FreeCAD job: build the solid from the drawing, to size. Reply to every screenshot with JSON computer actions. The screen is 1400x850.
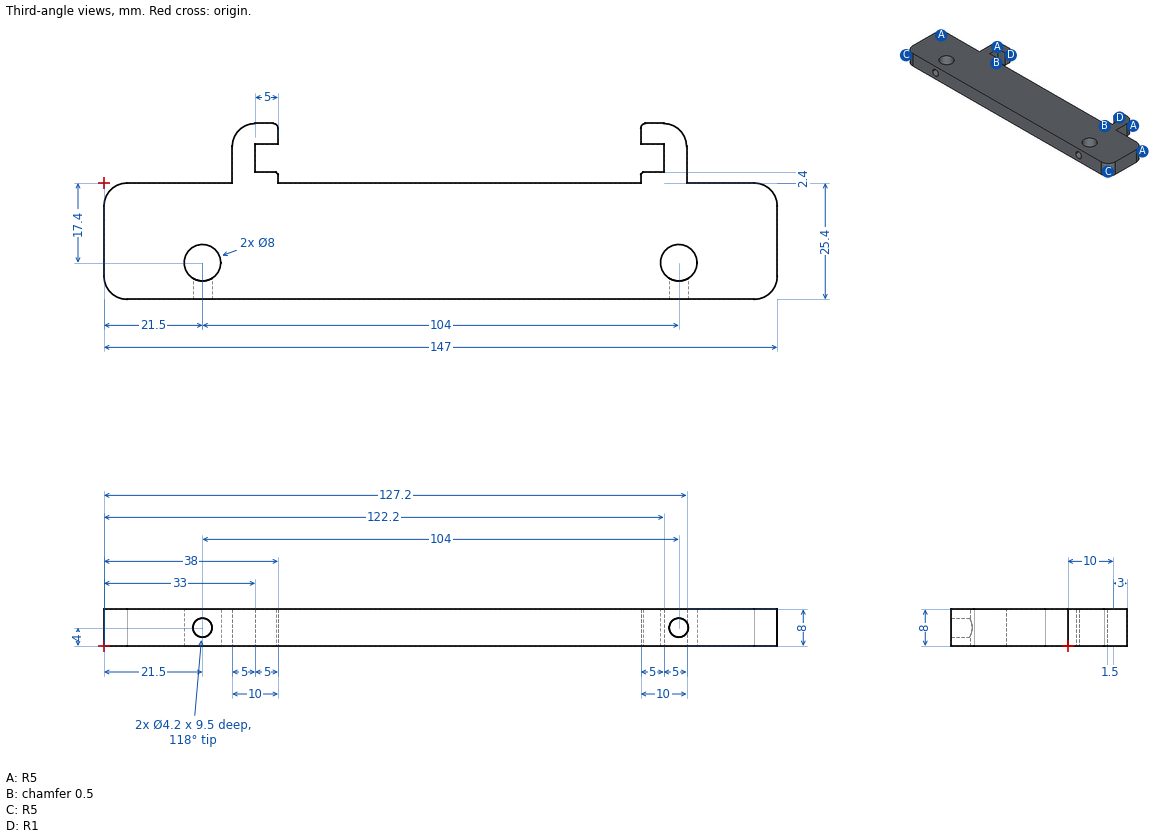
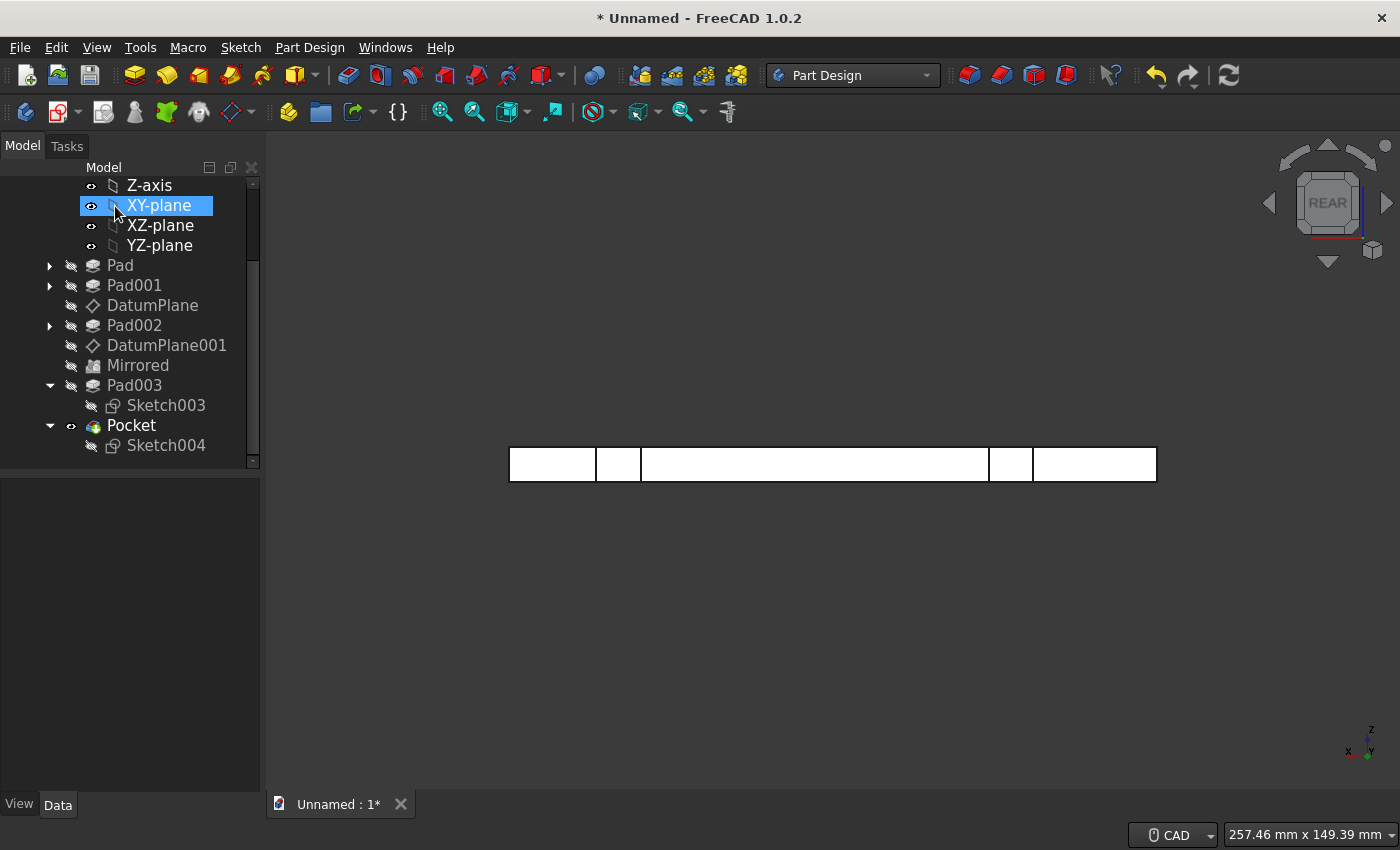
{"action": "left_click", "coordinate": [619, 463]}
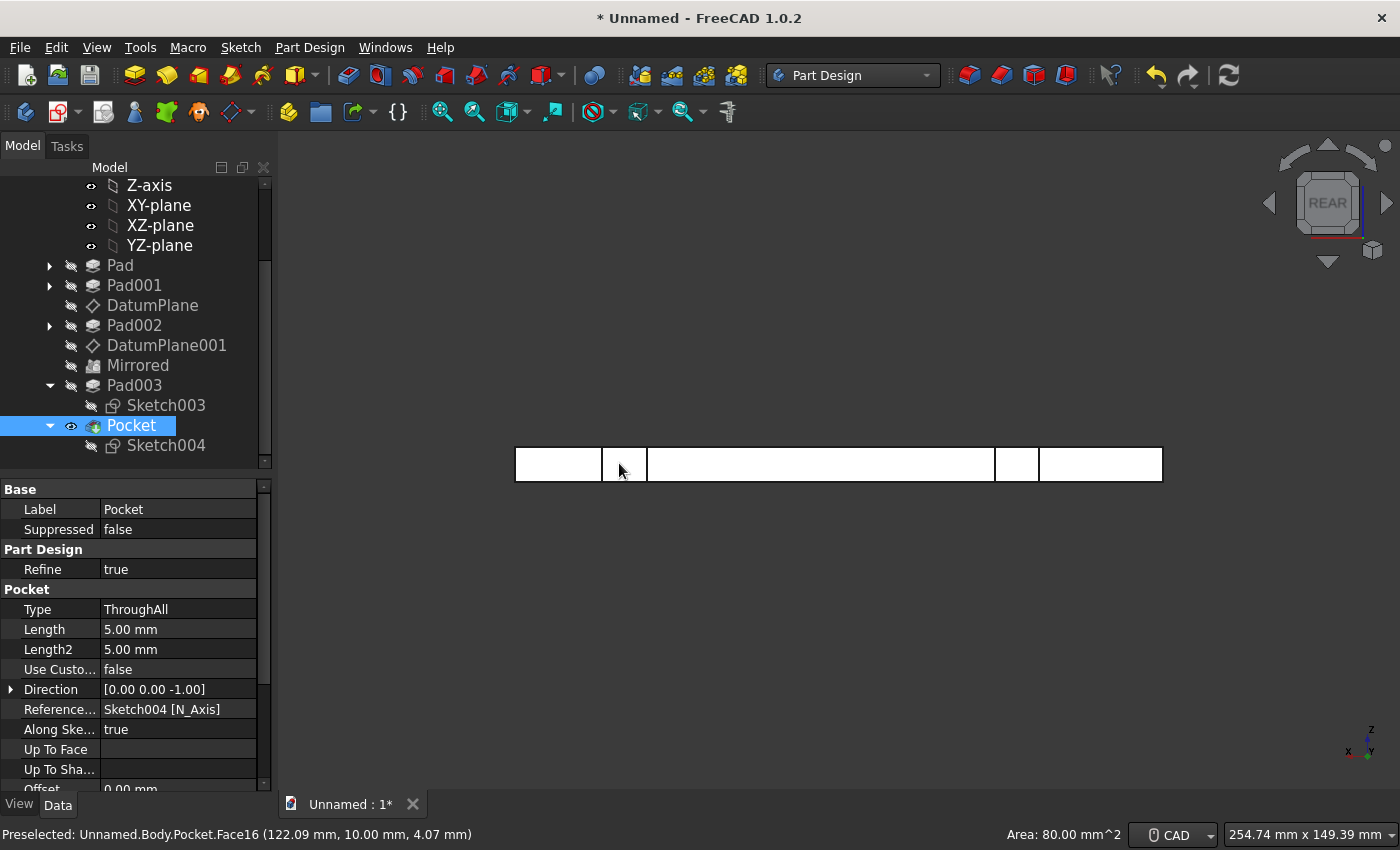
{"action": "left_click", "coordinate": [58, 112]}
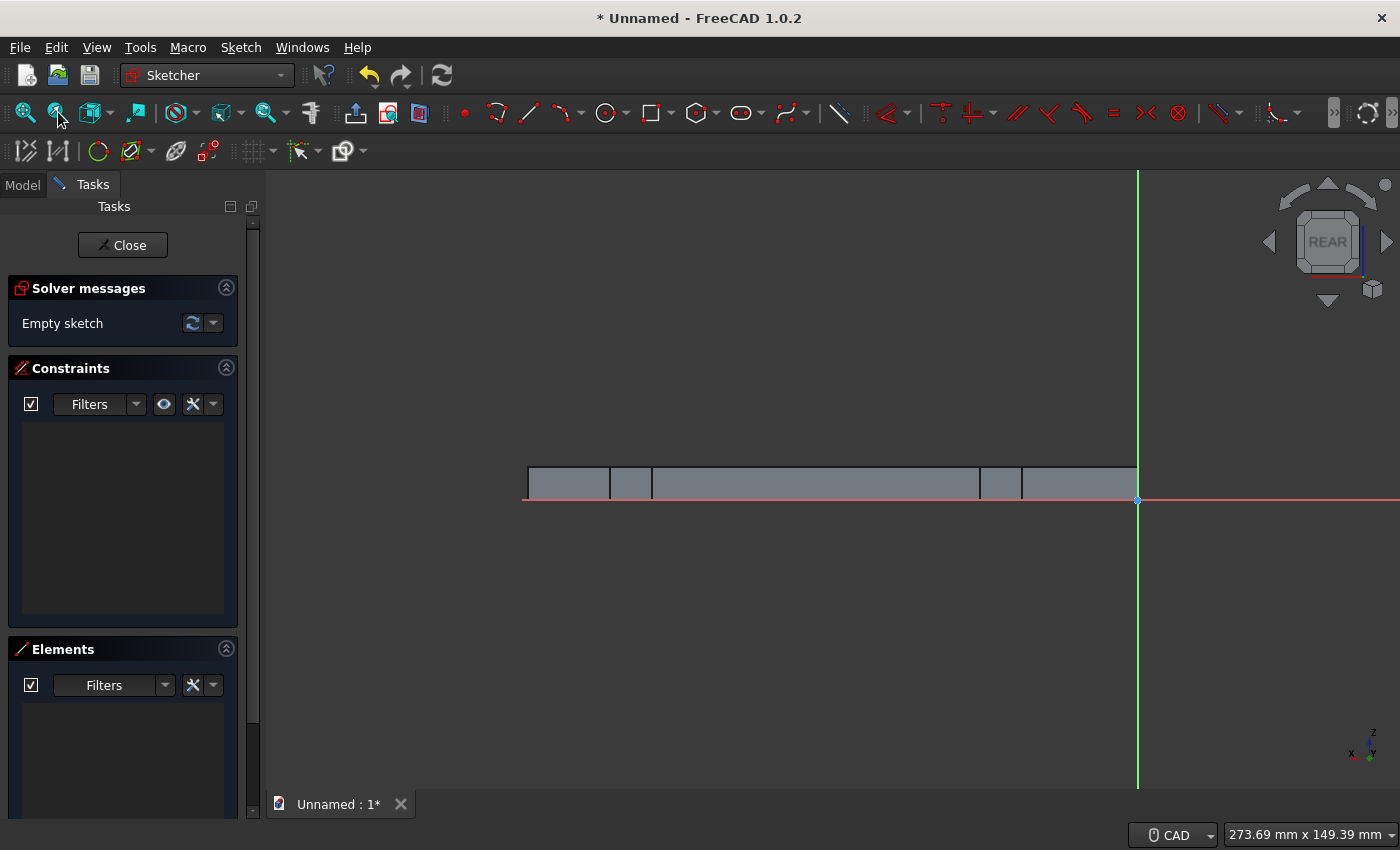
{"action": "key", "text": "g r"}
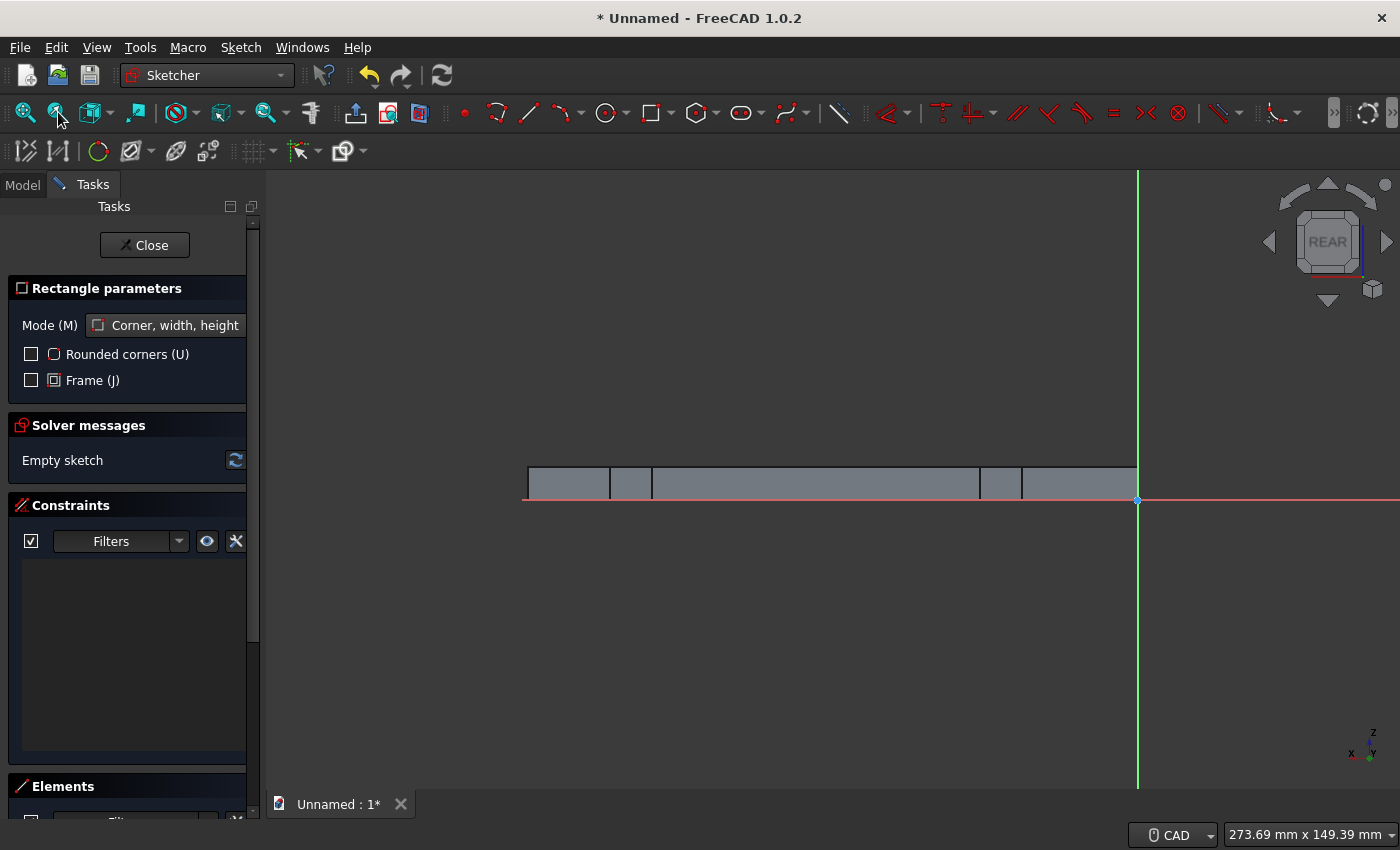
{"action": "left_click", "coordinate": [980, 467]}
{"action": "left_click", "coordinate": [1022, 500]}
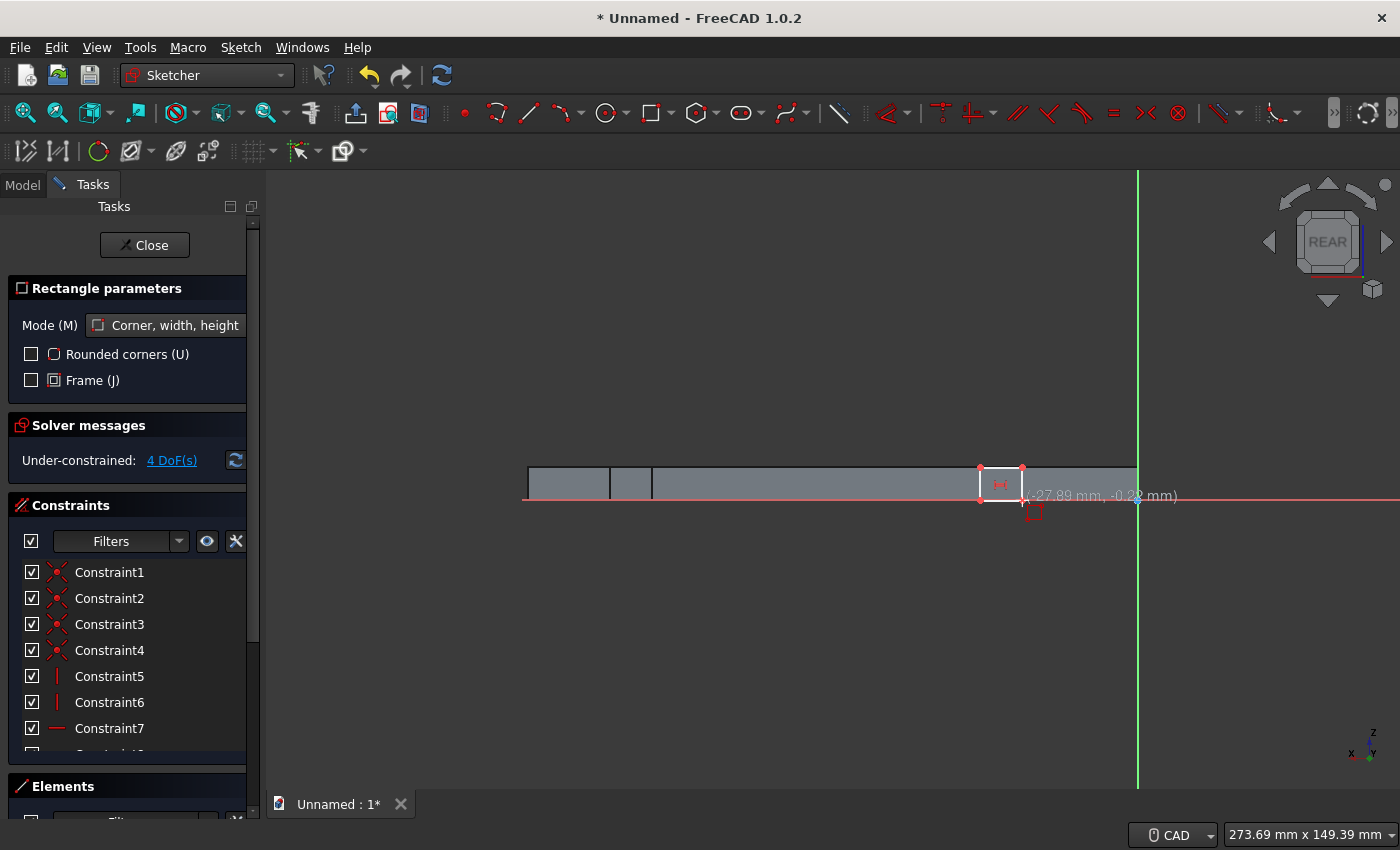
{"action": "left_click", "coordinate": [610, 467]}
{"action": "left_click", "coordinate": [652, 500]}
{"action": "key", "text": "Escape"}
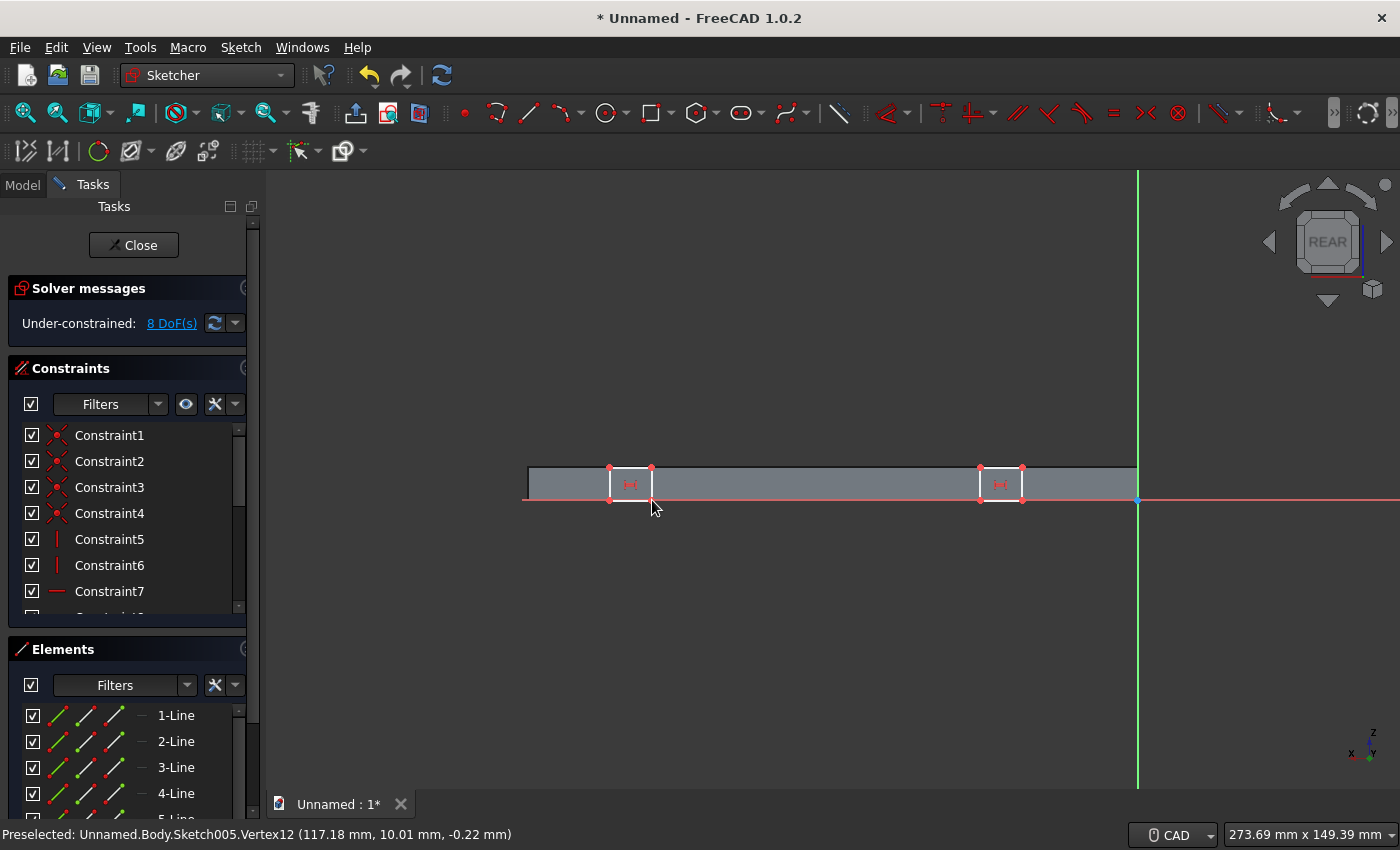
{"action": "left_click", "coordinate": [980, 501]}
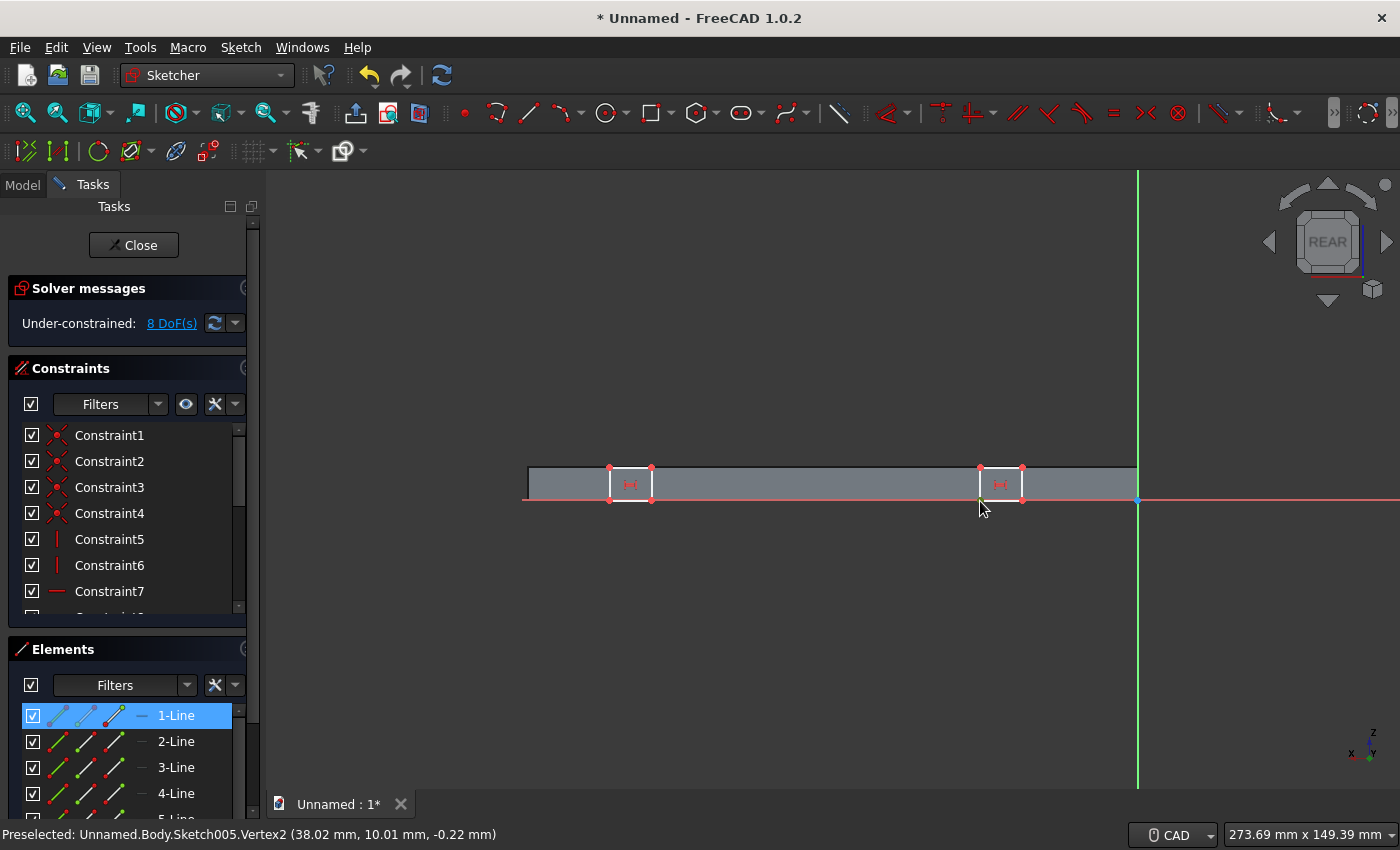
{"action": "left_click", "coordinate": [563, 500]}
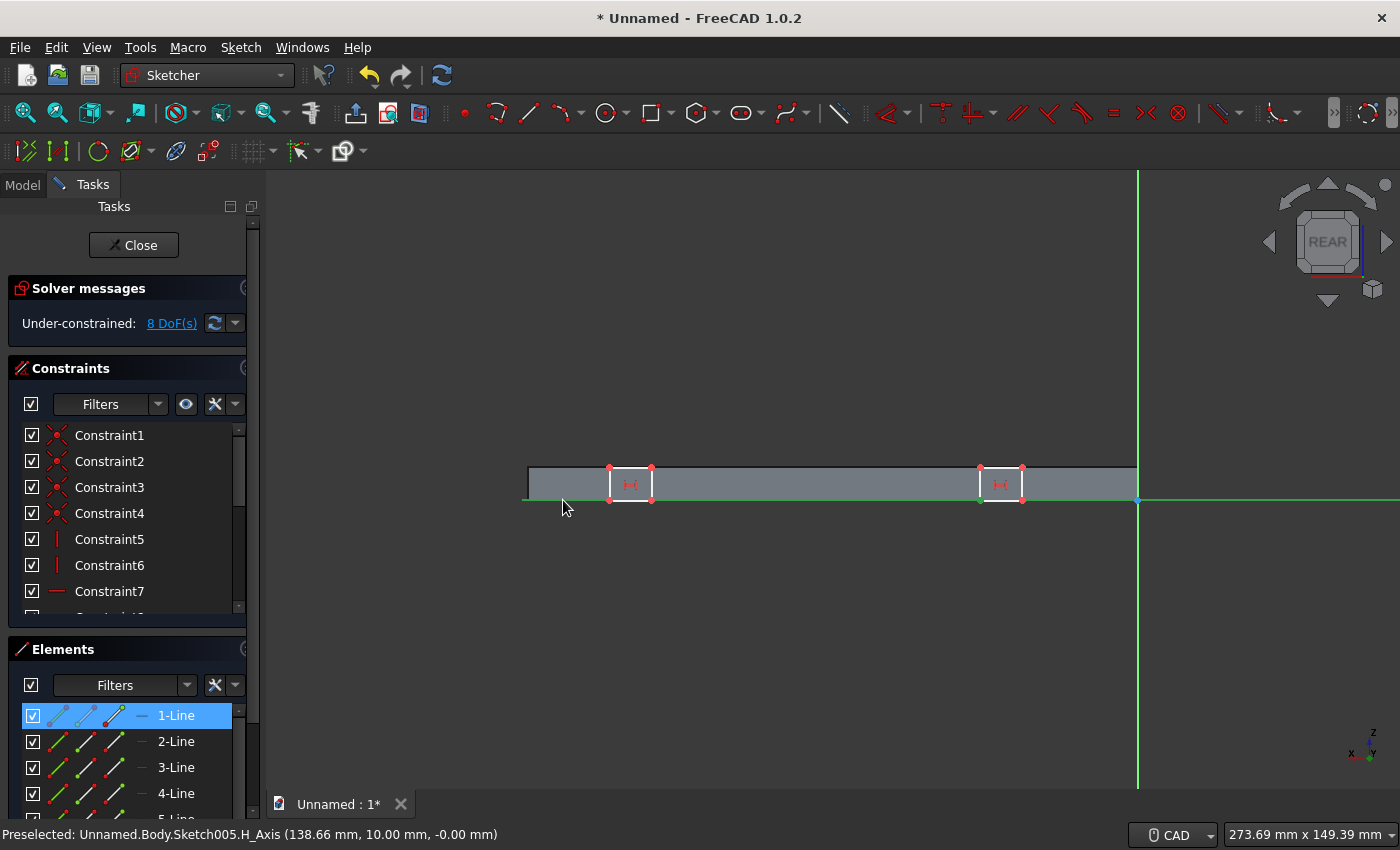
{"action": "left_click", "coordinate": [942, 114]}